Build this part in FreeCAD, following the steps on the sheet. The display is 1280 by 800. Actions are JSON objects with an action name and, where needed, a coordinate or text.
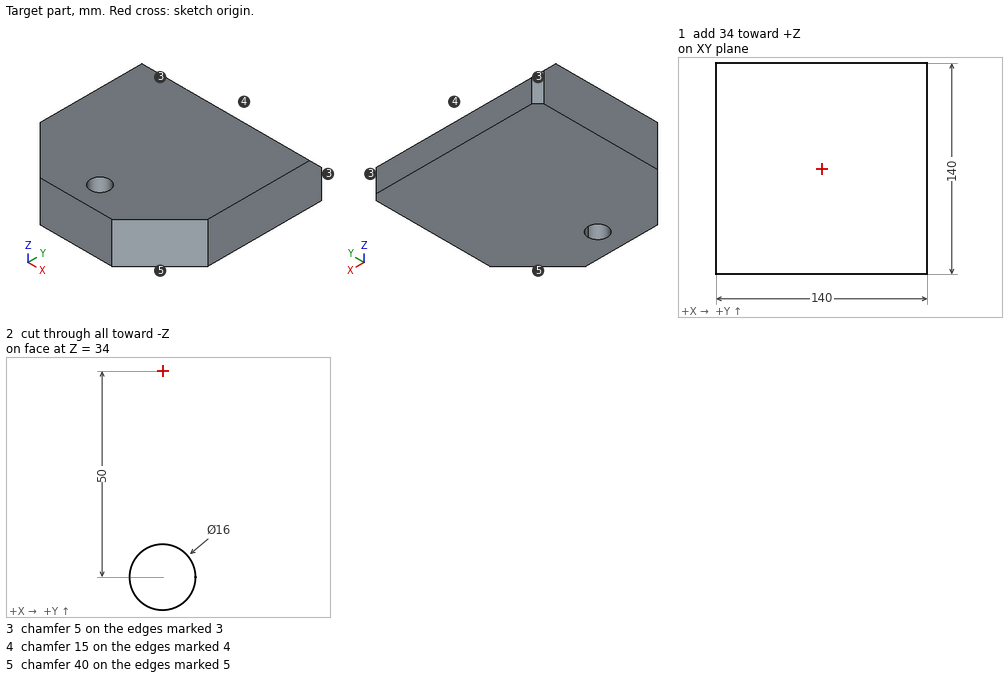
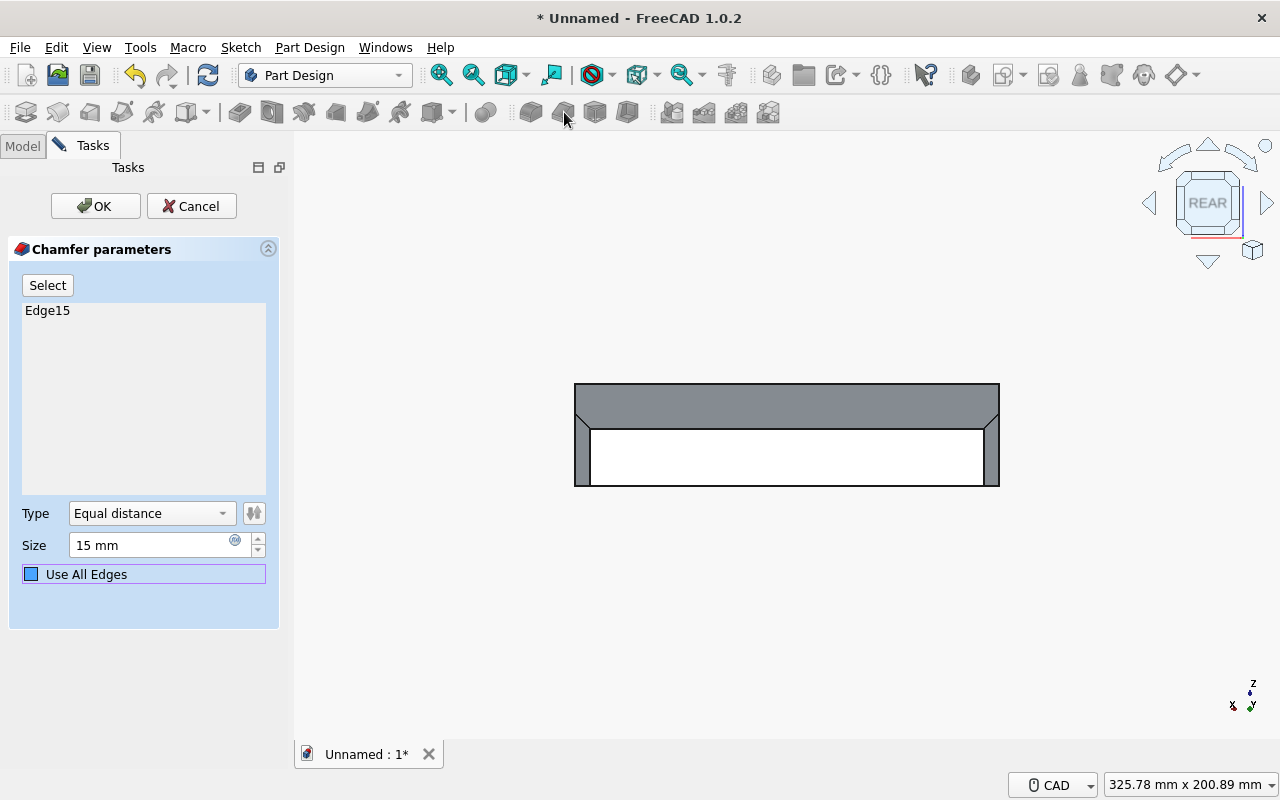
{"action": "left_click", "coordinate": [96, 206]}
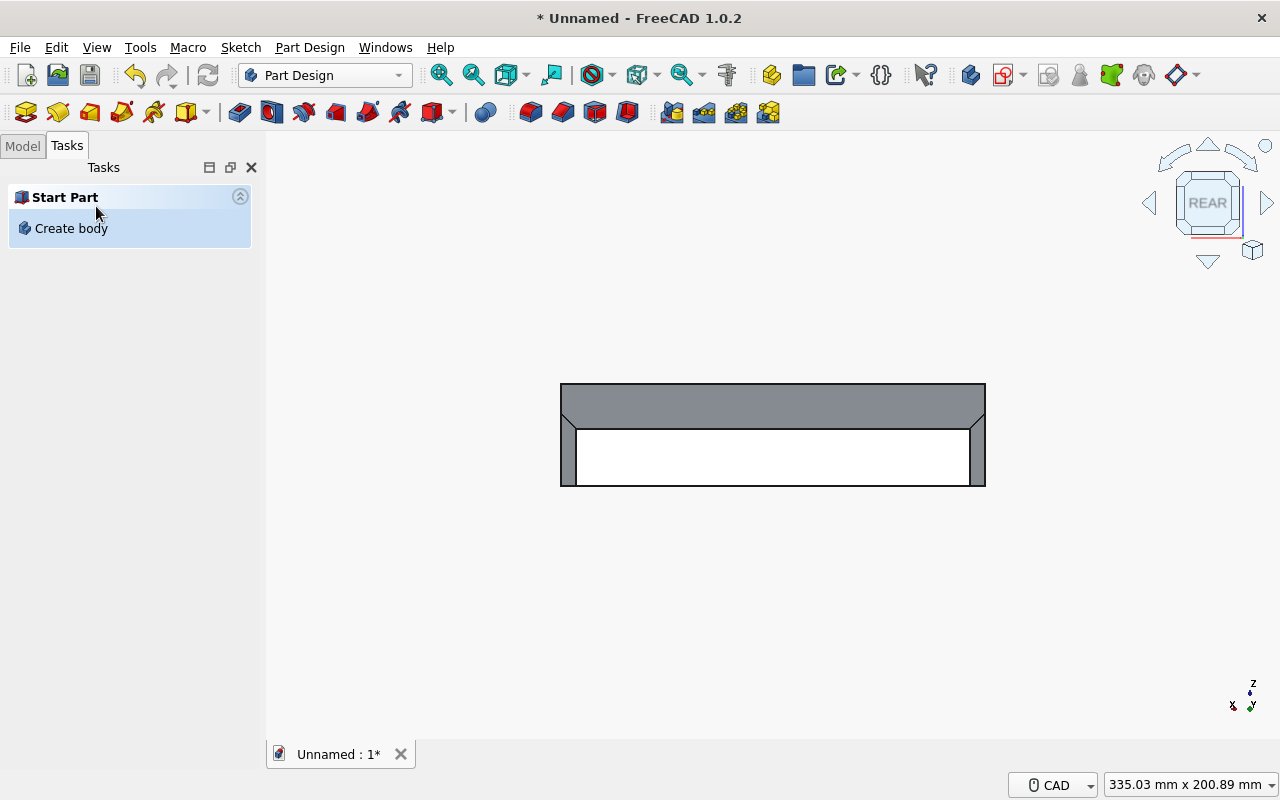
{"action": "key", "text": "v f"}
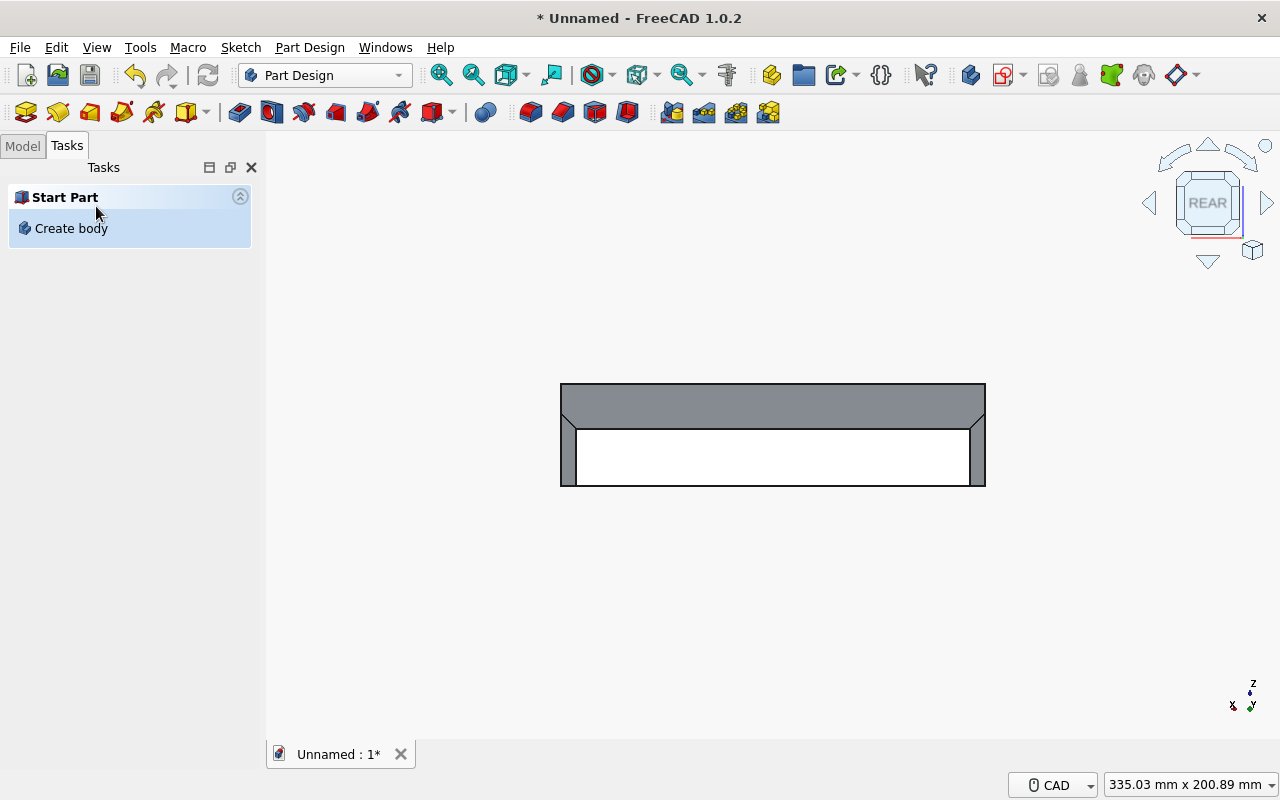
{"action": "key", "text": "0"}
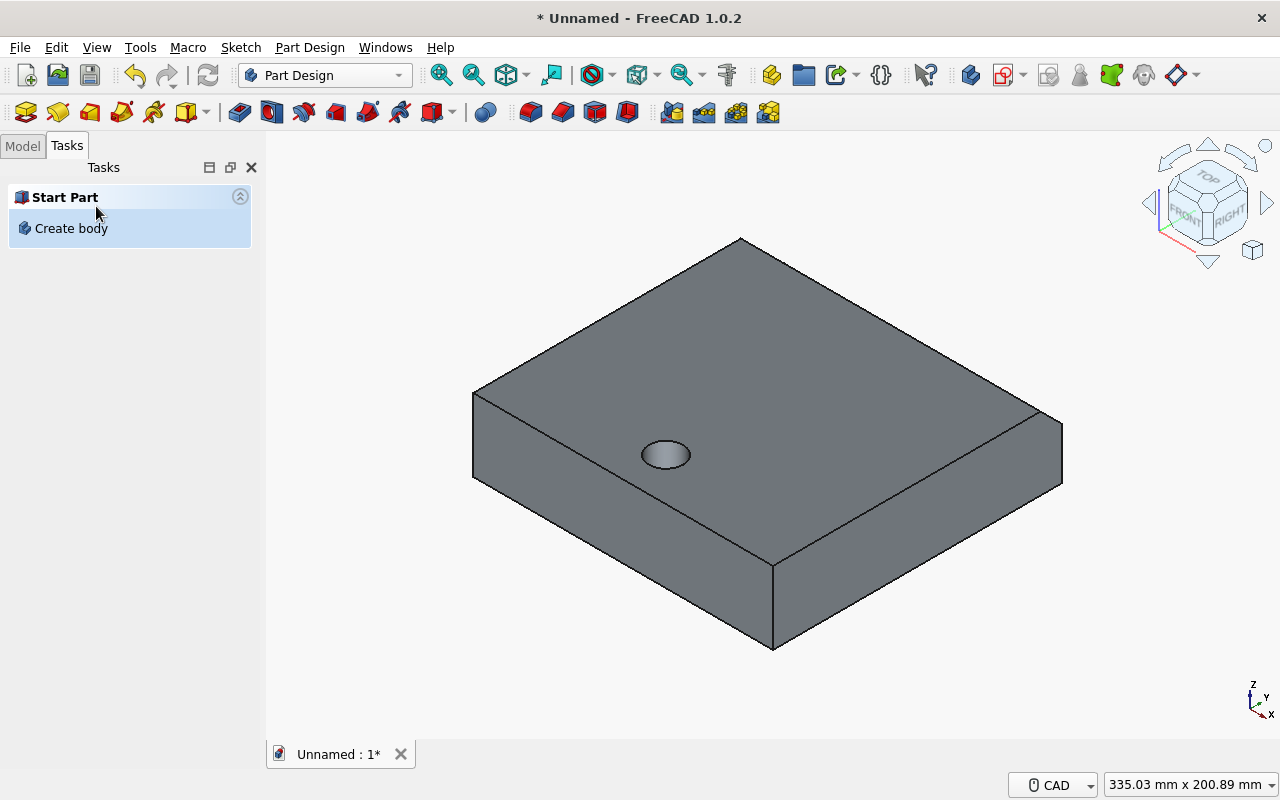
{"action": "left_click", "coordinate": [773, 607]}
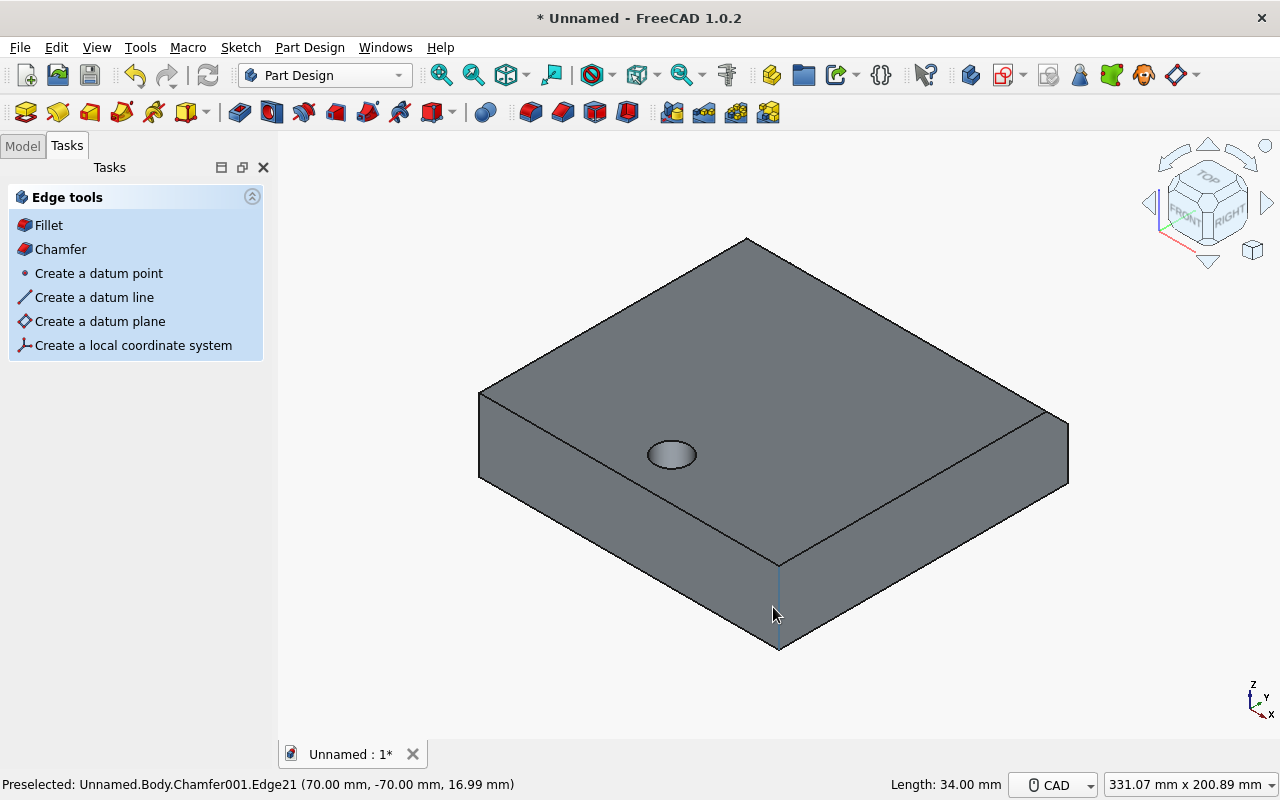
{"action": "key", "text": "2"}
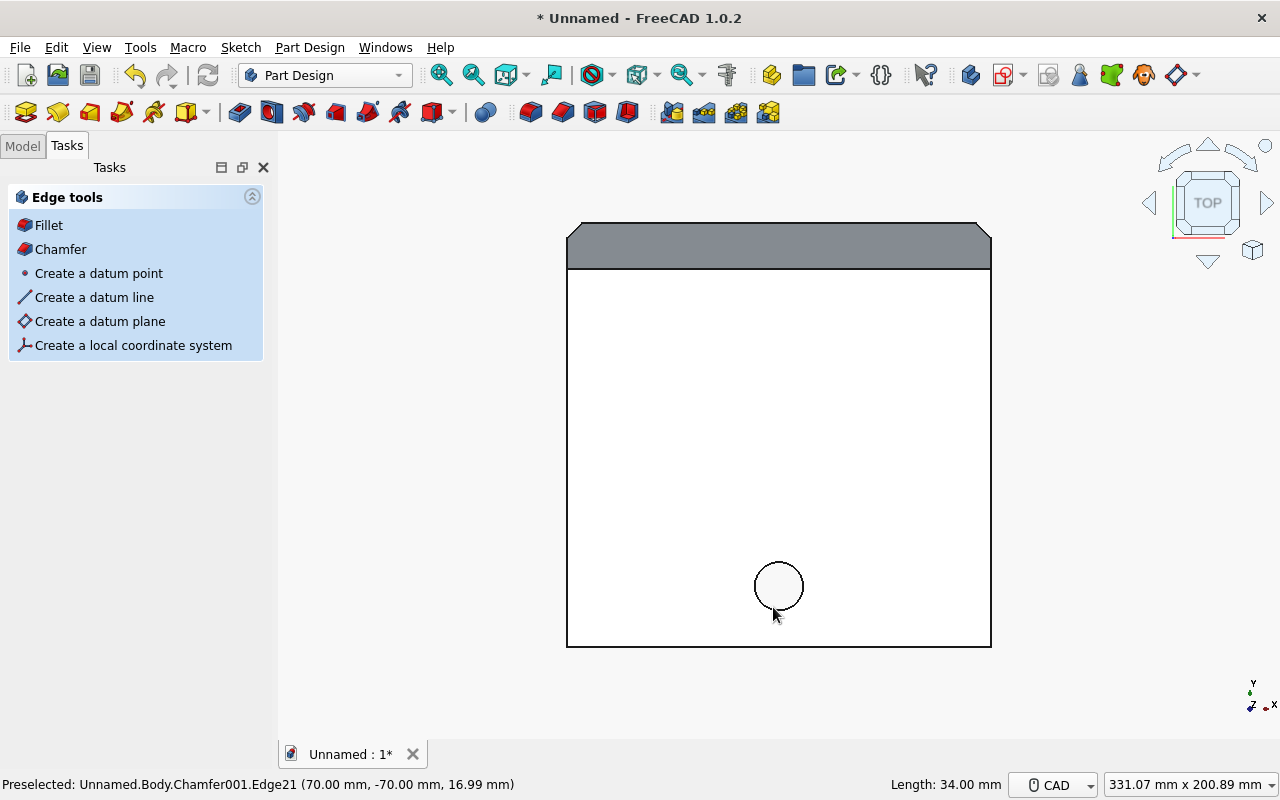
{"action": "key", "text": "1"}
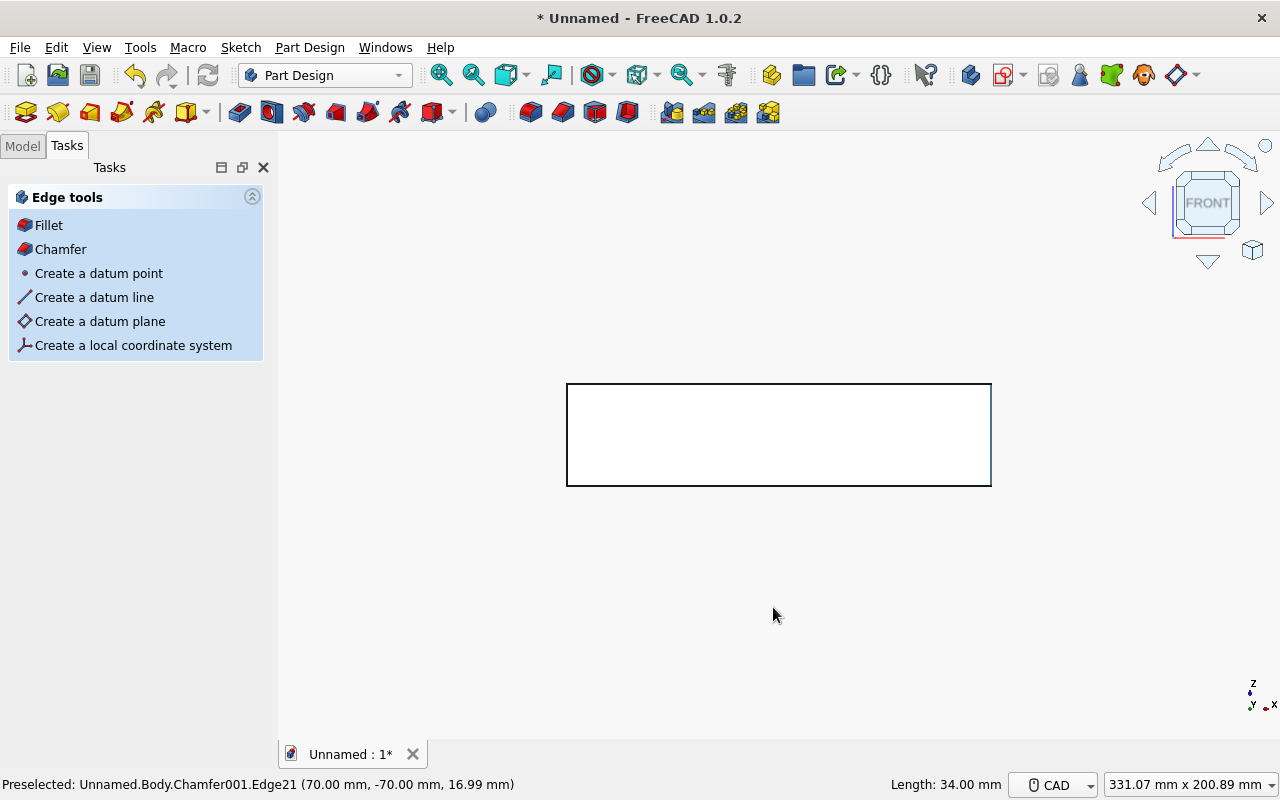
{"action": "left_click", "coordinate": [442, 76]}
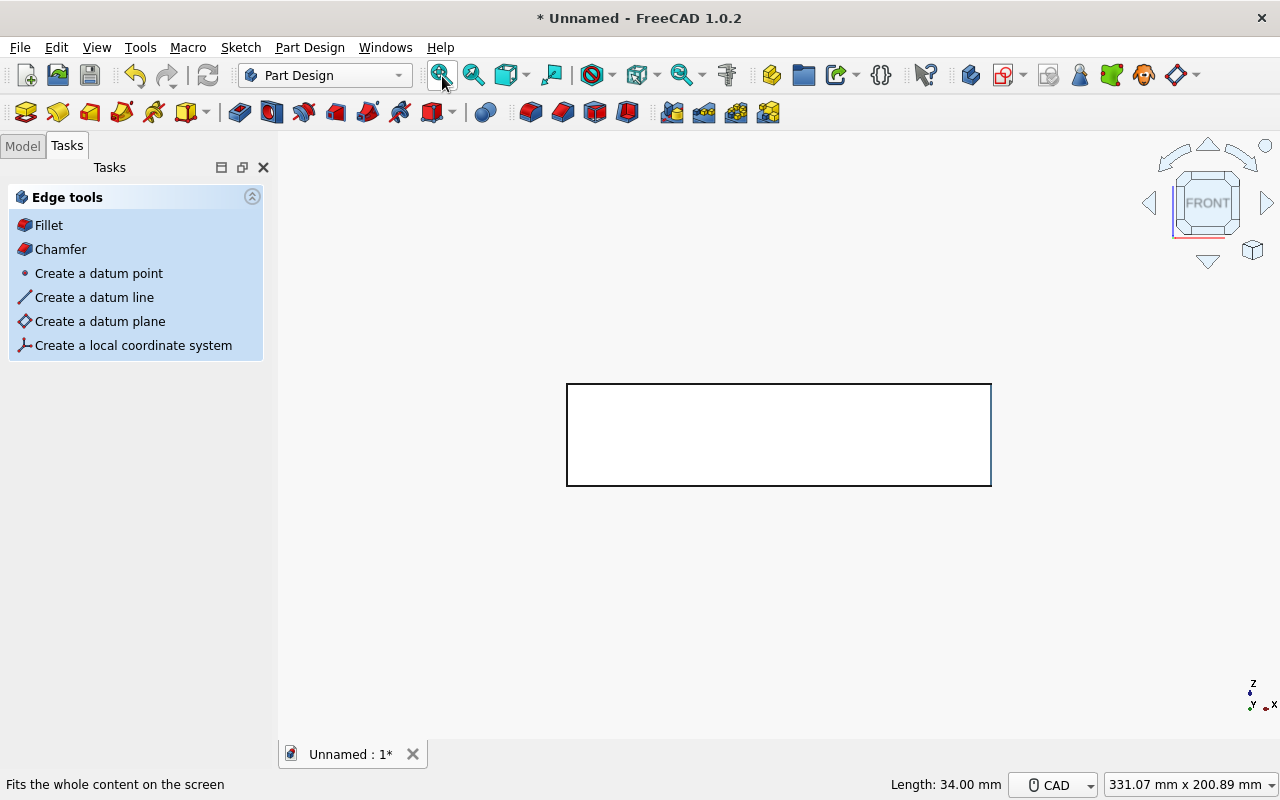
{"action": "left_click", "coordinate": [567, 434], "text": "ctrl"}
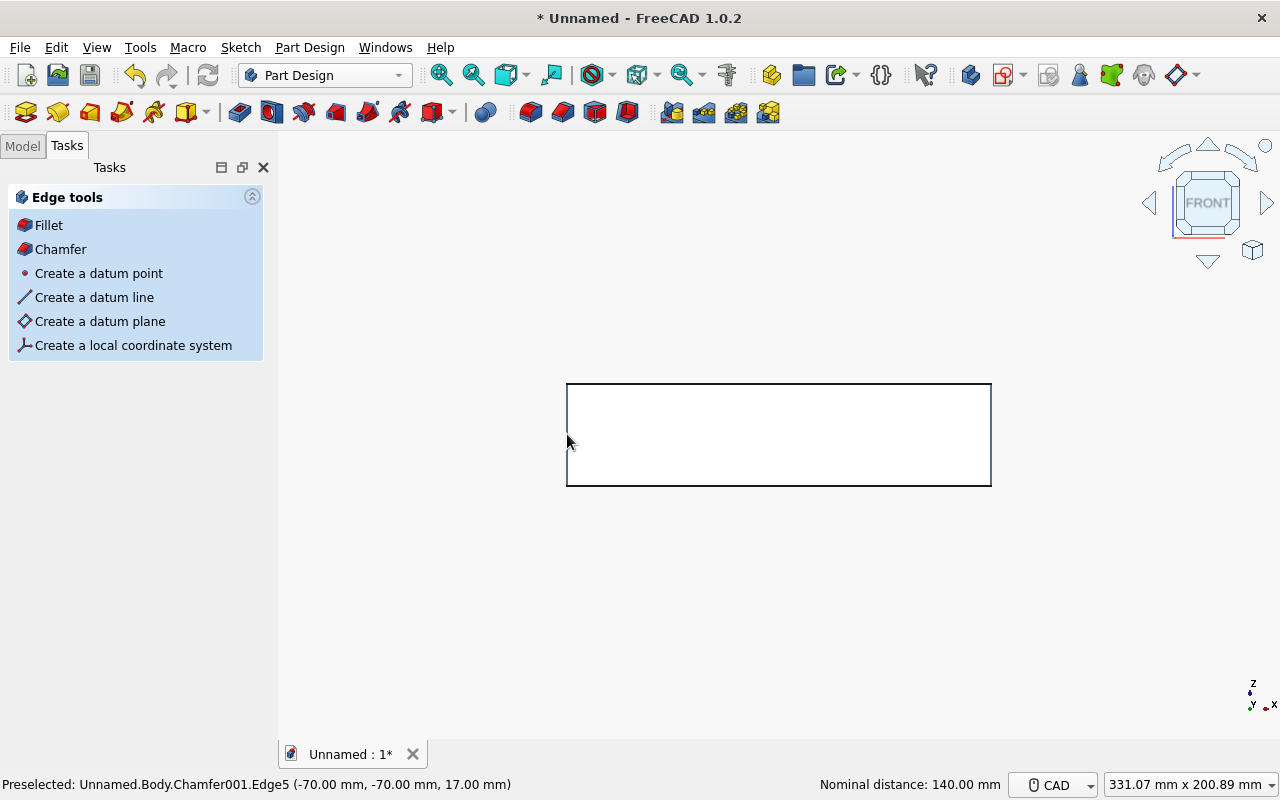
{"action": "left_click", "coordinate": [564, 112]}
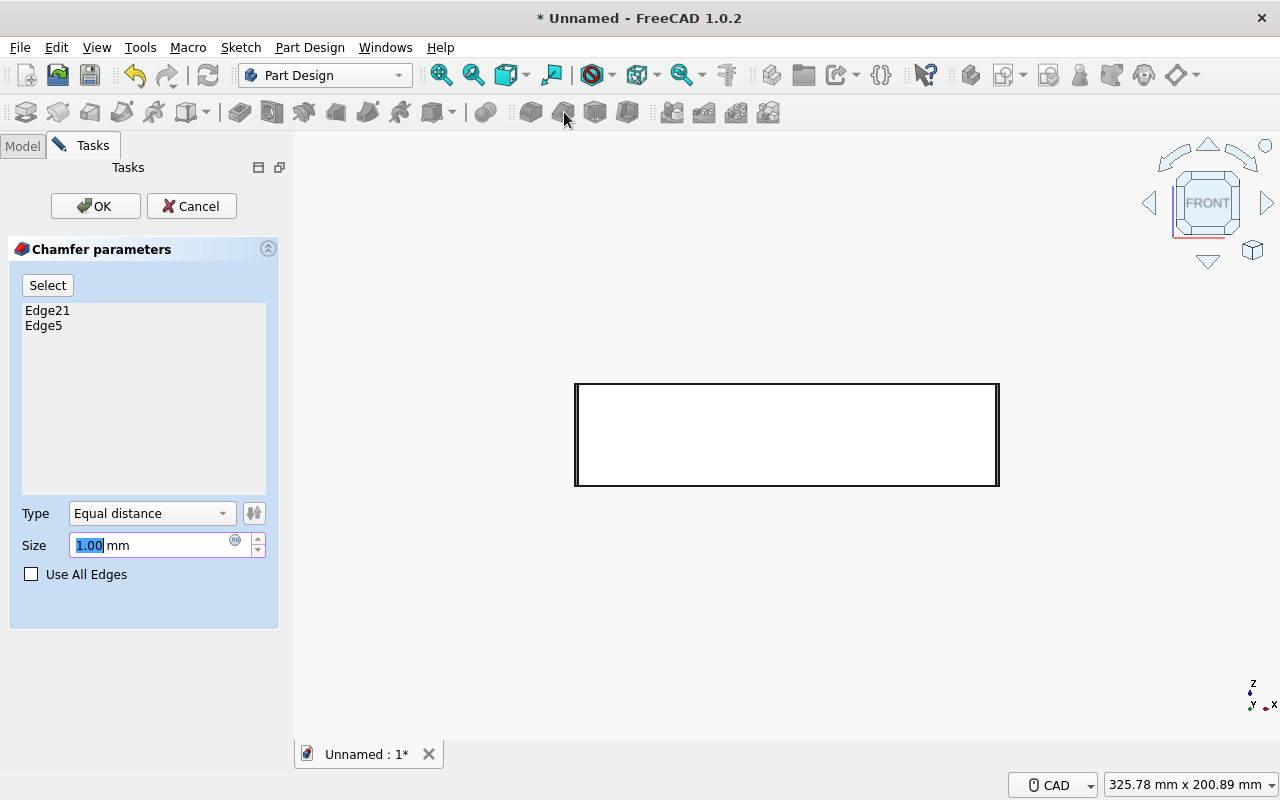
{"action": "type", "text": "40"}
{"action": "key", "text": "Tab"}